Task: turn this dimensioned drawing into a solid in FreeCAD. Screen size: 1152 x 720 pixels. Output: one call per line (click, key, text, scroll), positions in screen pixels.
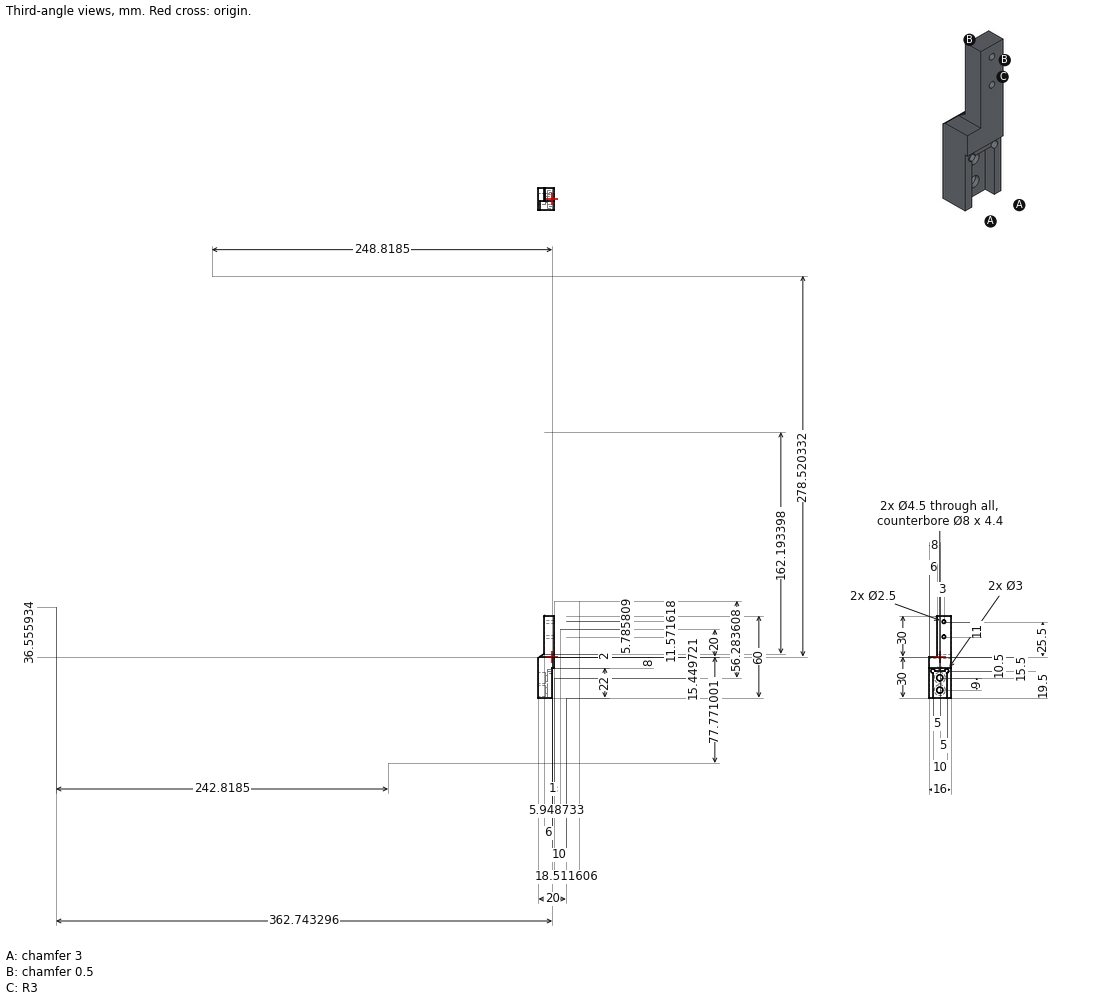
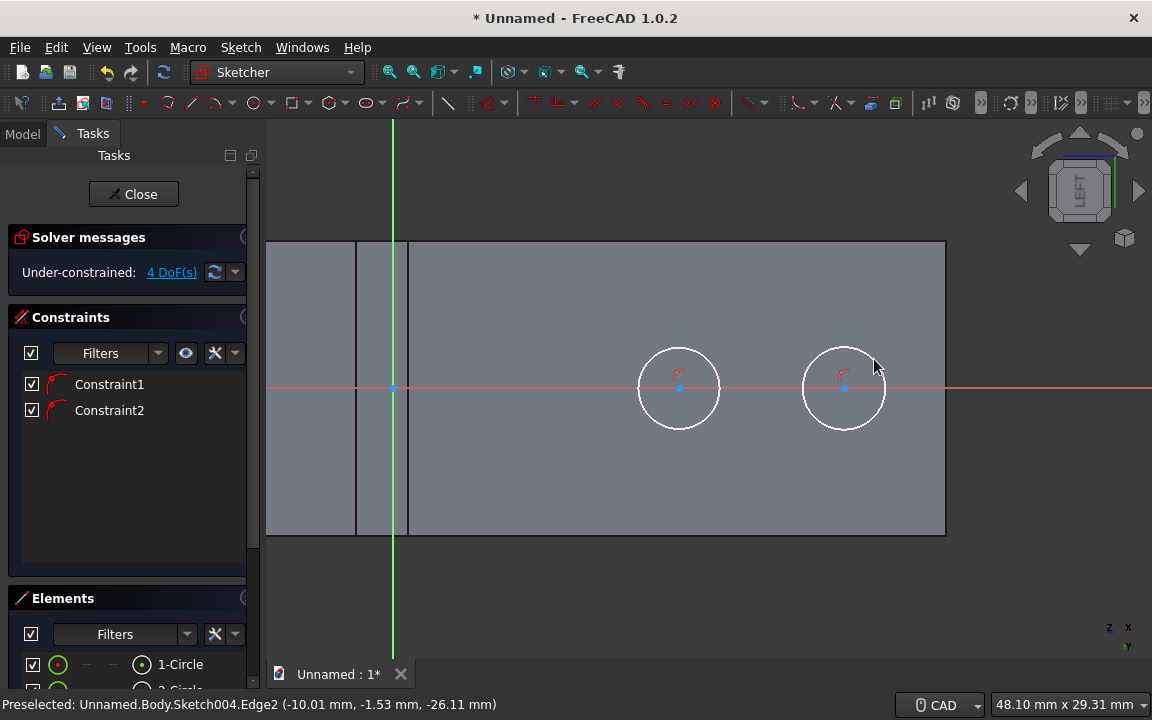
click(708, 360)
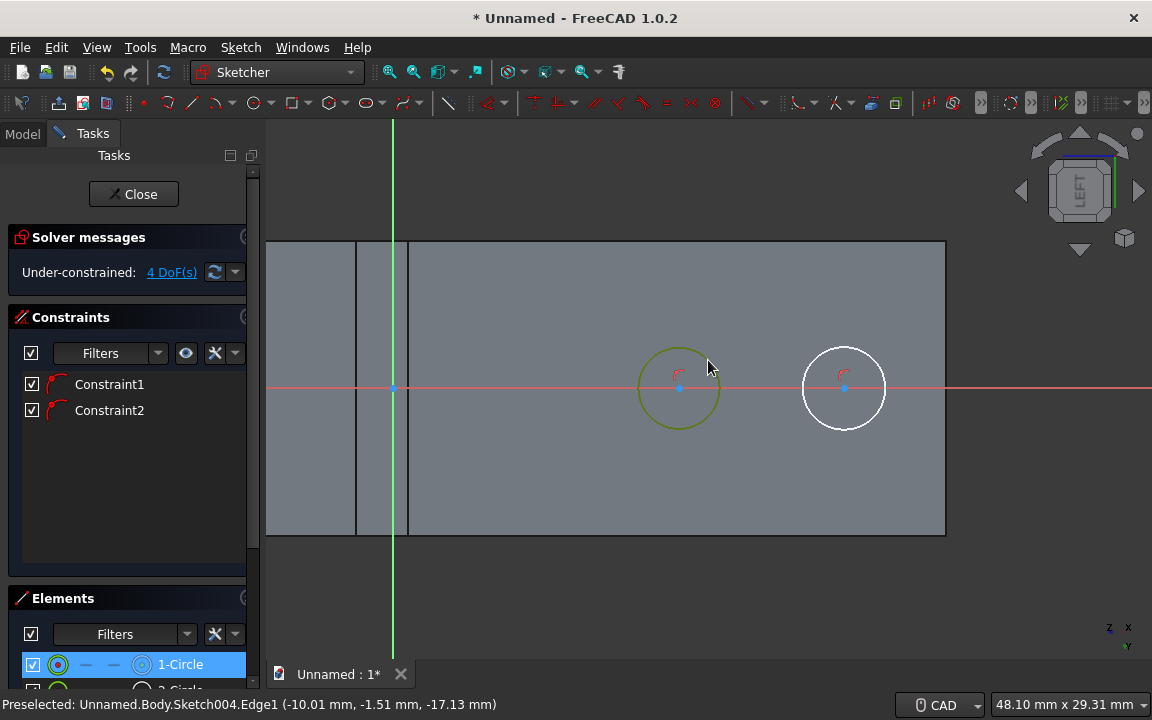
click(873, 359)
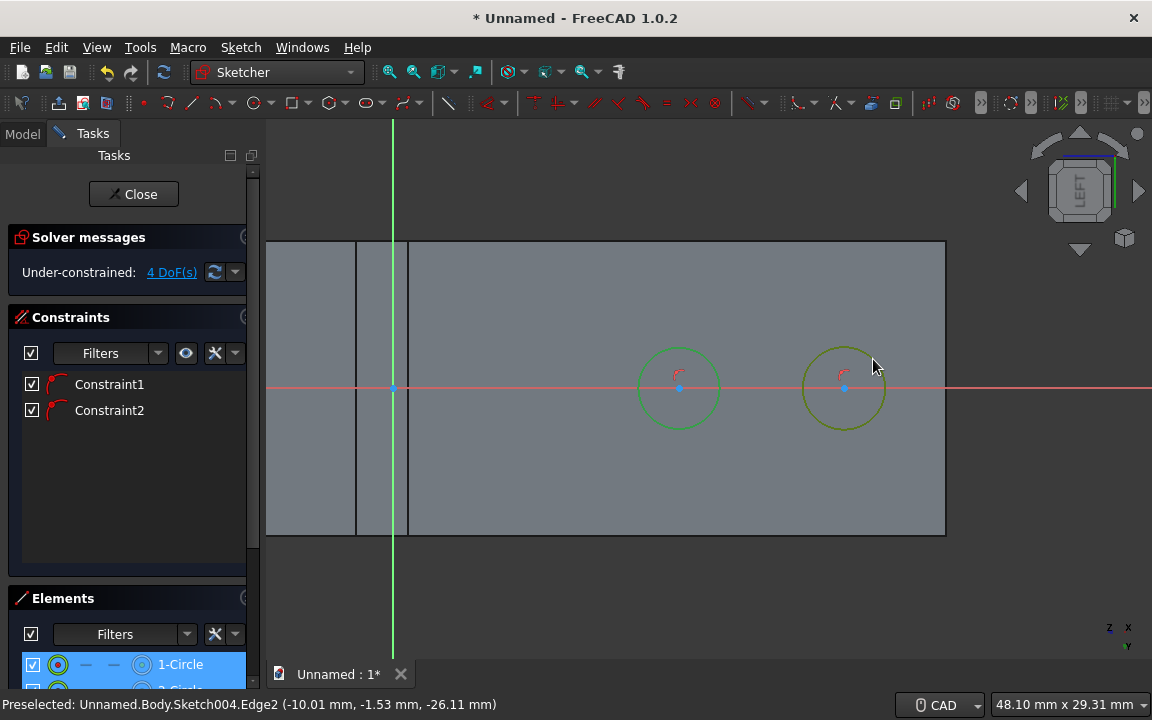
click(668, 104)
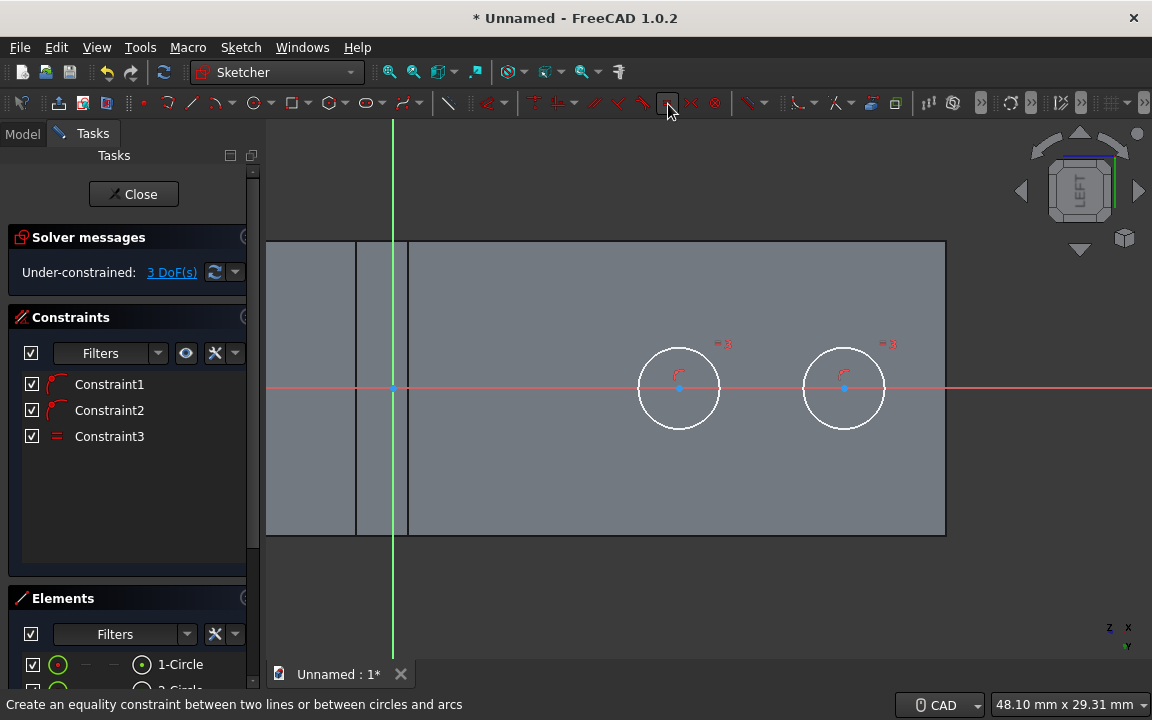
key(d)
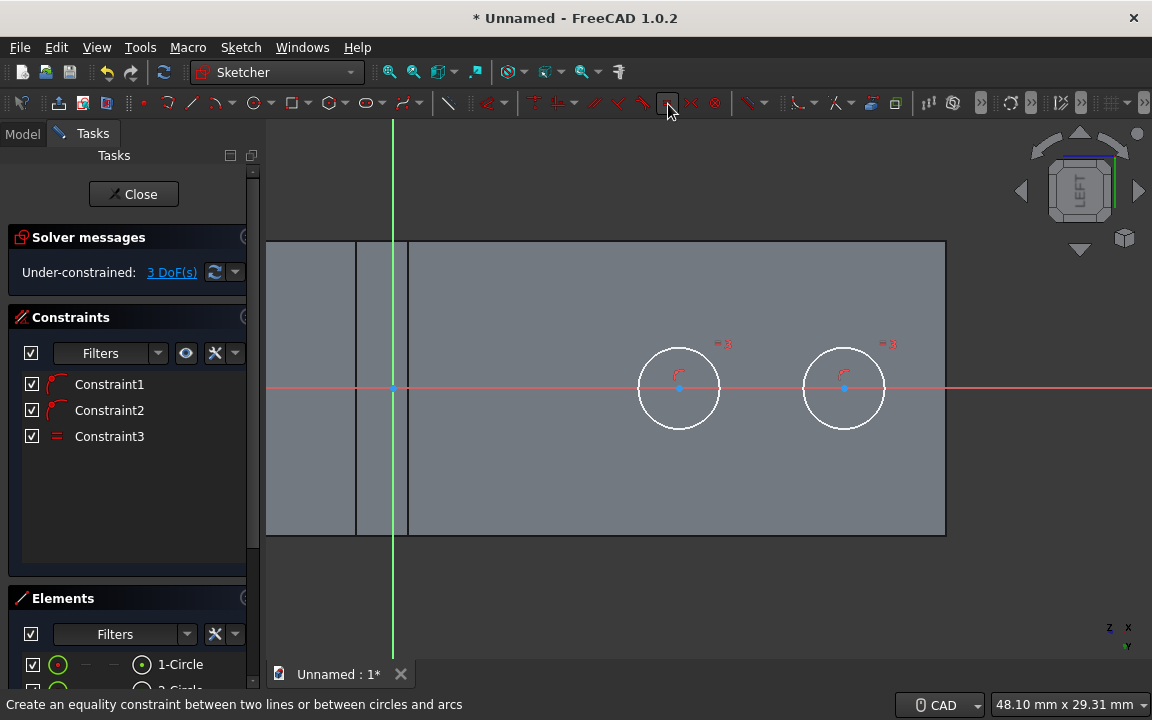
click(708, 360)
click(731, 338)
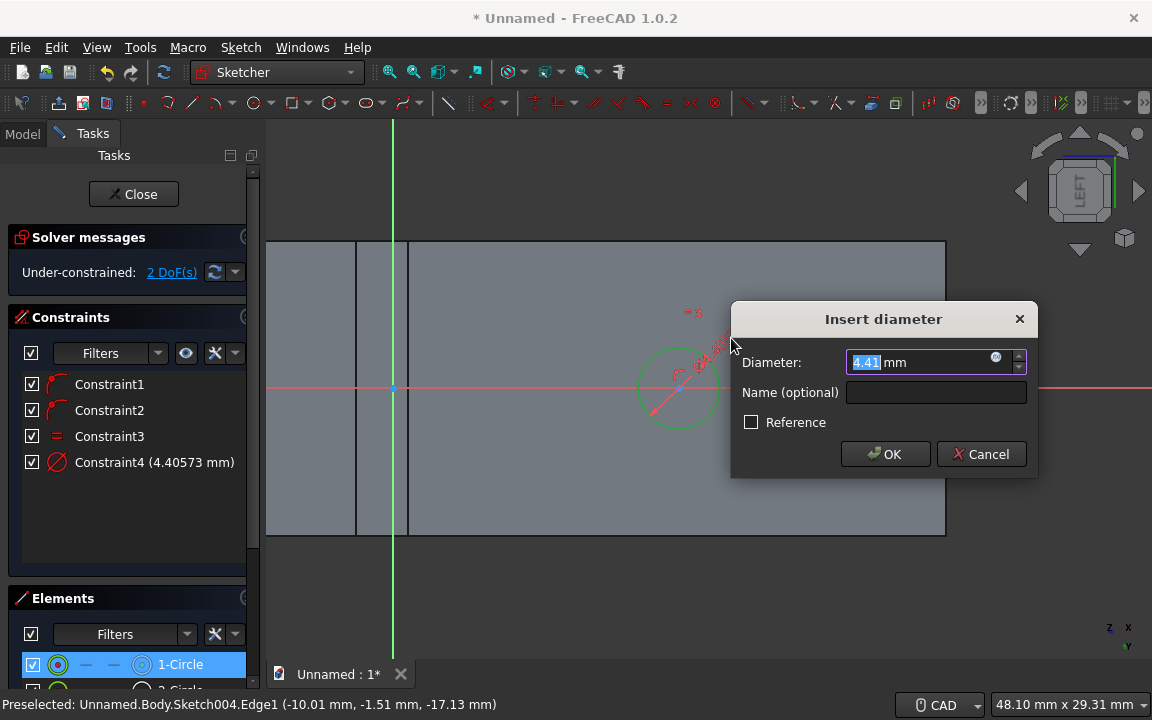
text(4.5)
key(Return)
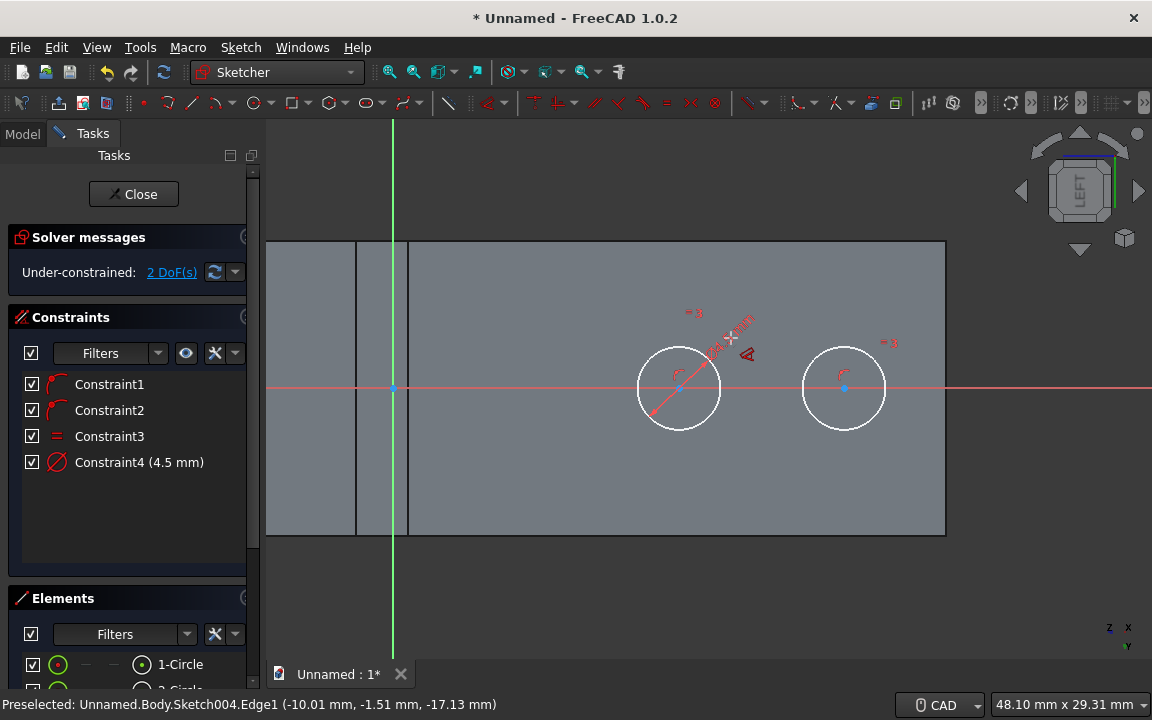
click(679, 388)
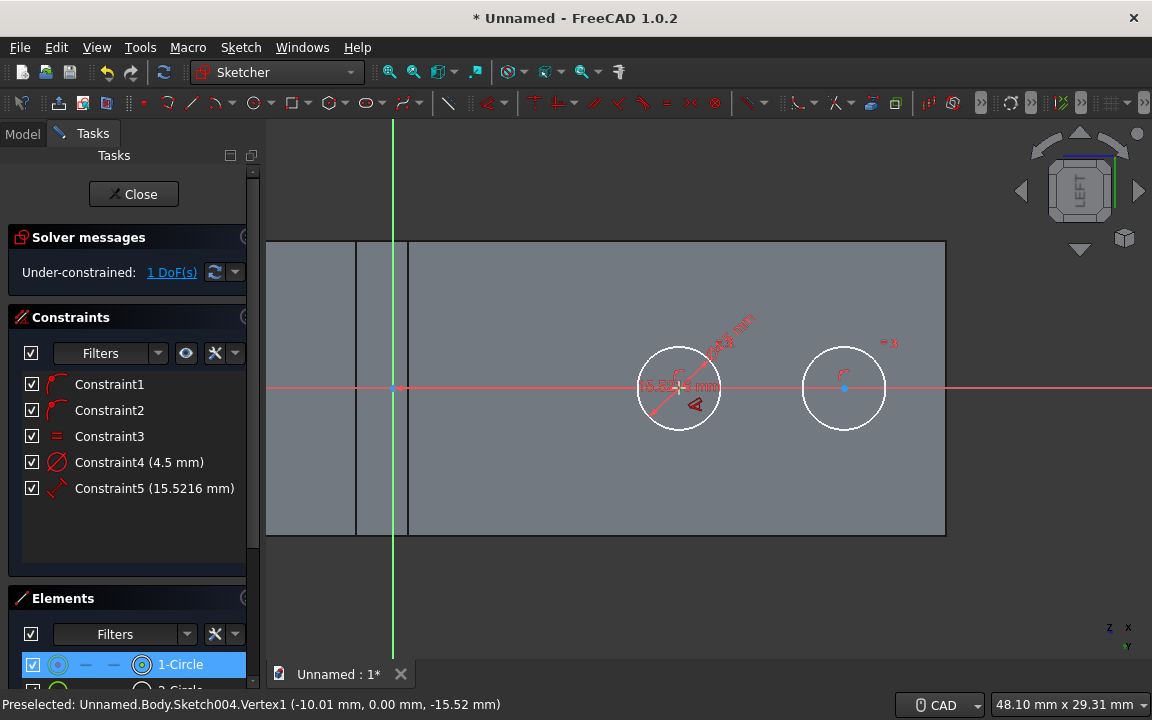
click(844, 388)
click(761, 422)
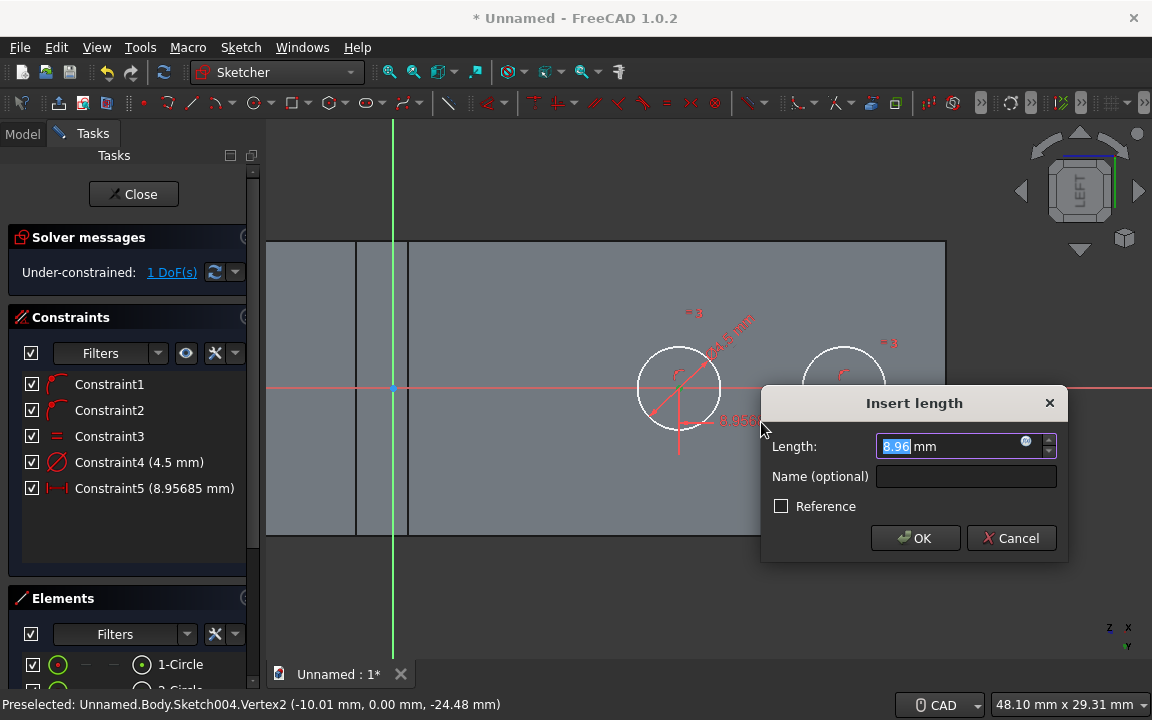
text(9)
key(Return)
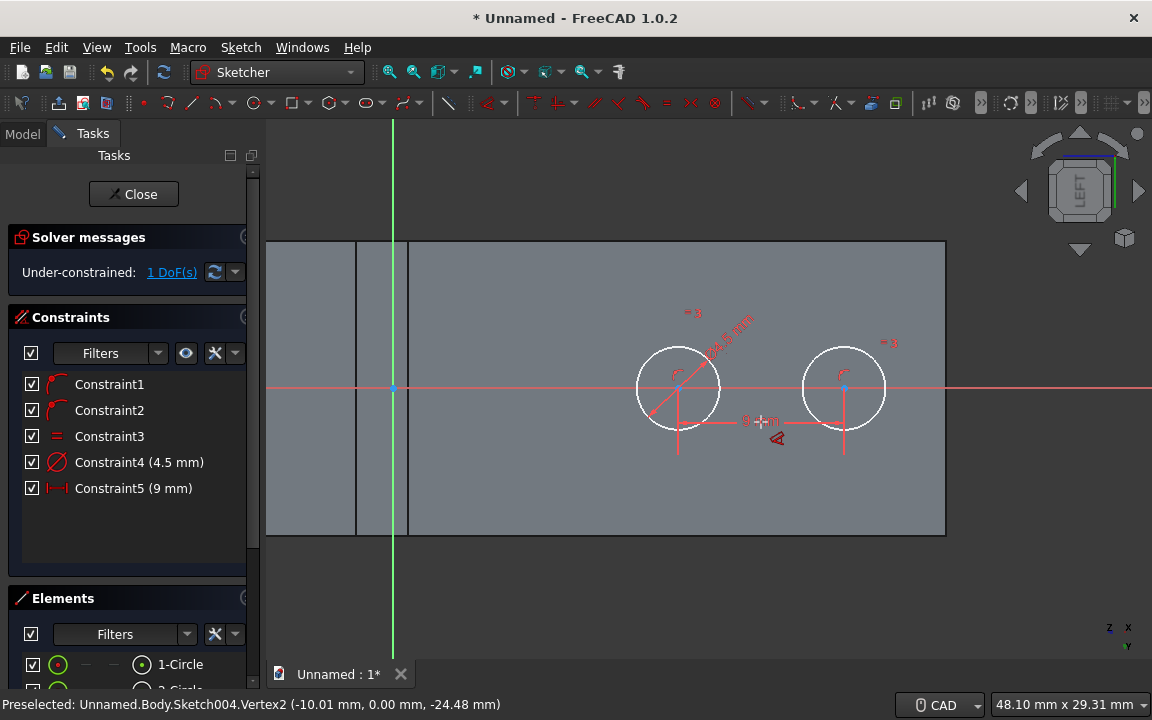
click(678, 388)
click(536, 422)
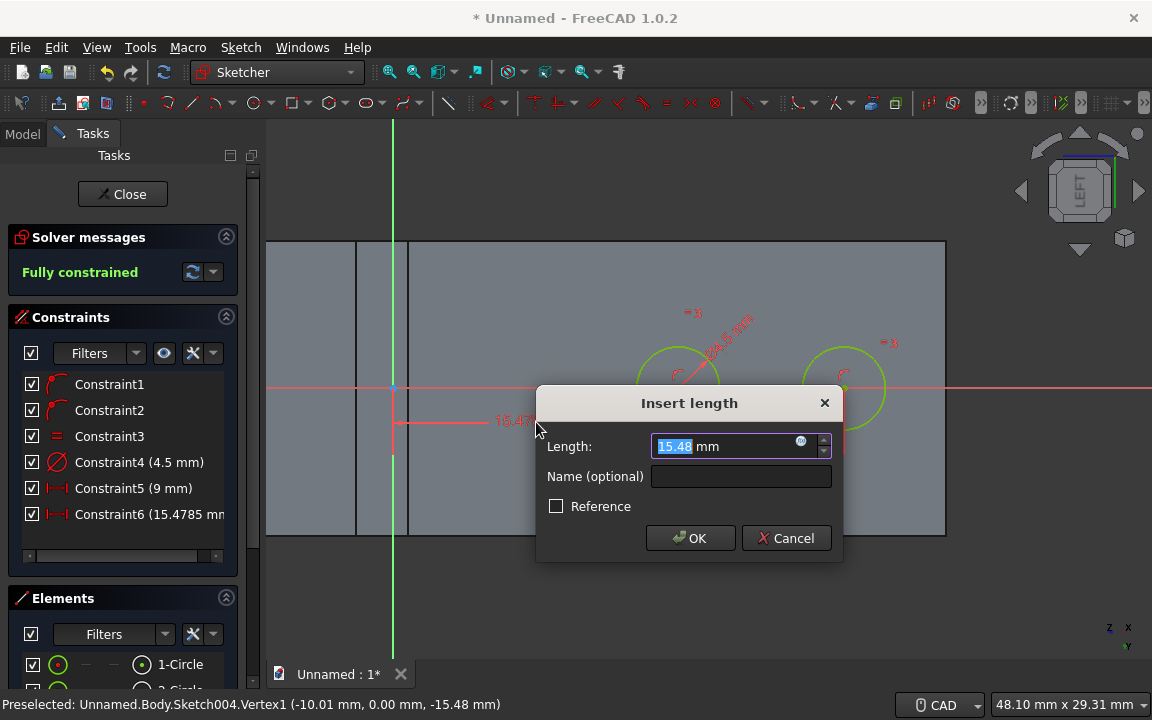
text(15.5)
key(Return)
key(Escape)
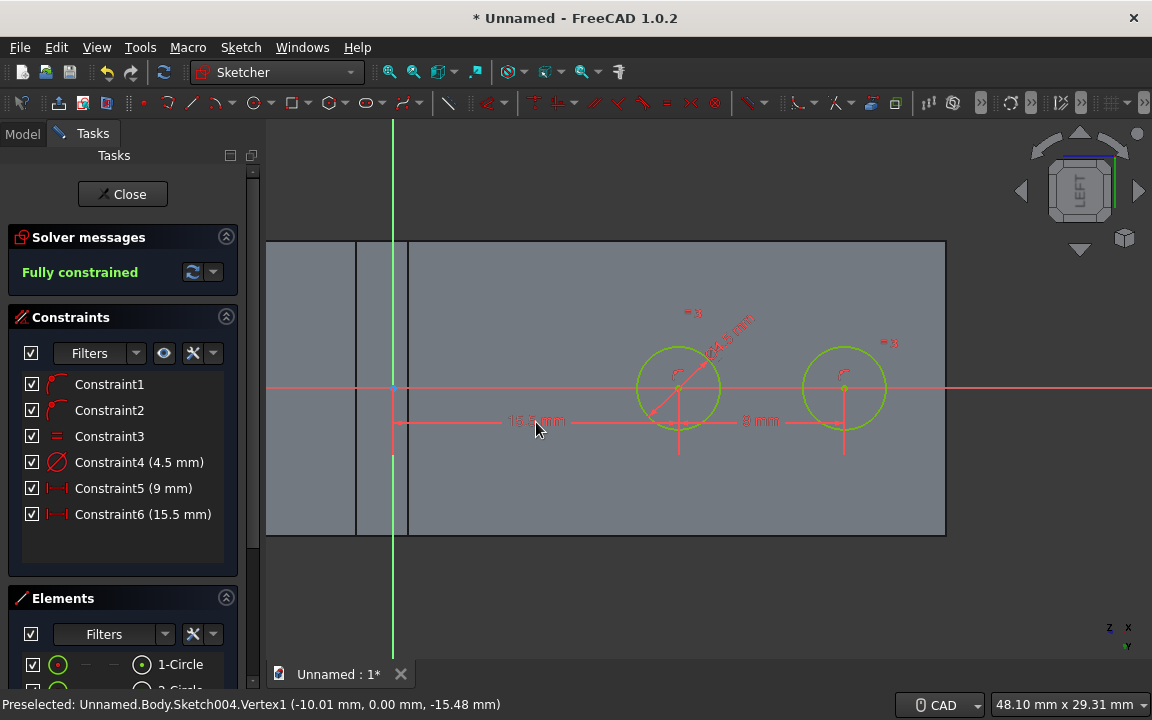
click(123, 194)